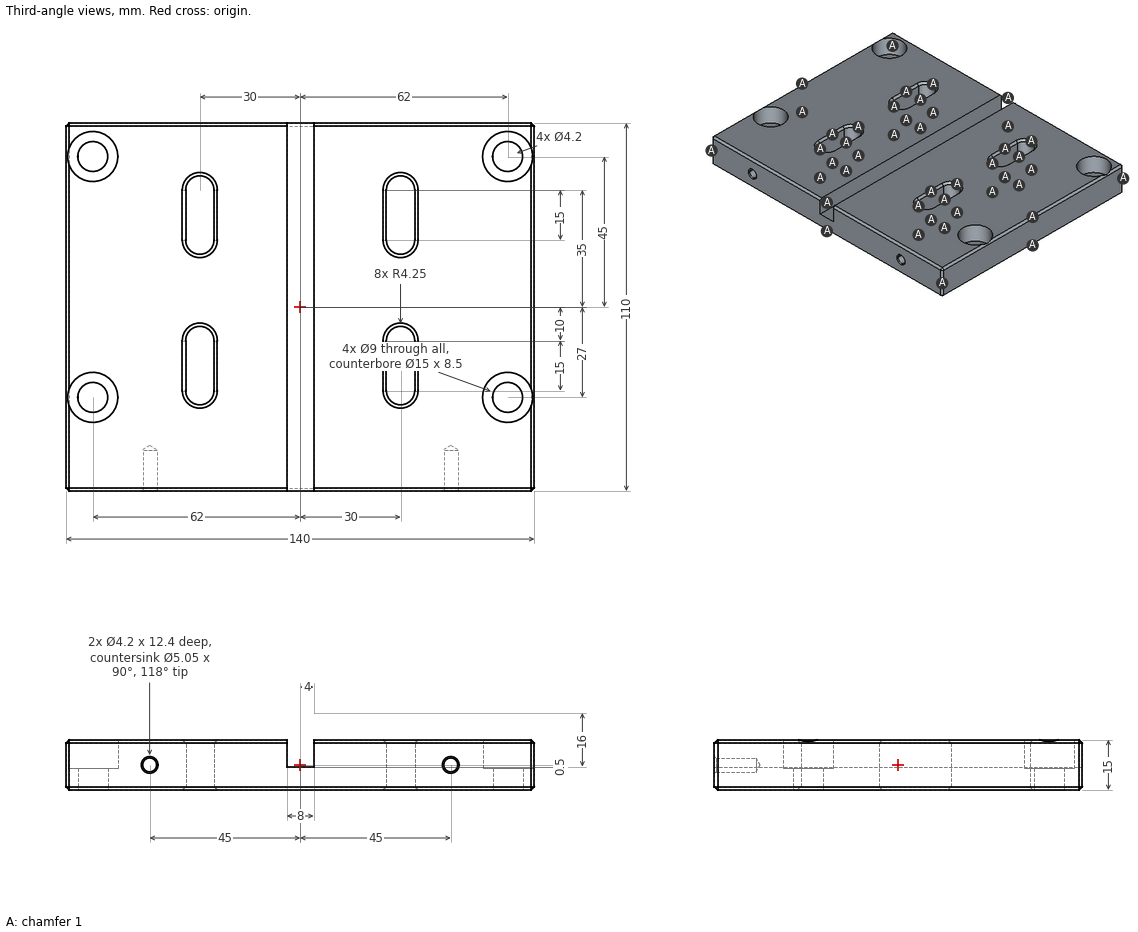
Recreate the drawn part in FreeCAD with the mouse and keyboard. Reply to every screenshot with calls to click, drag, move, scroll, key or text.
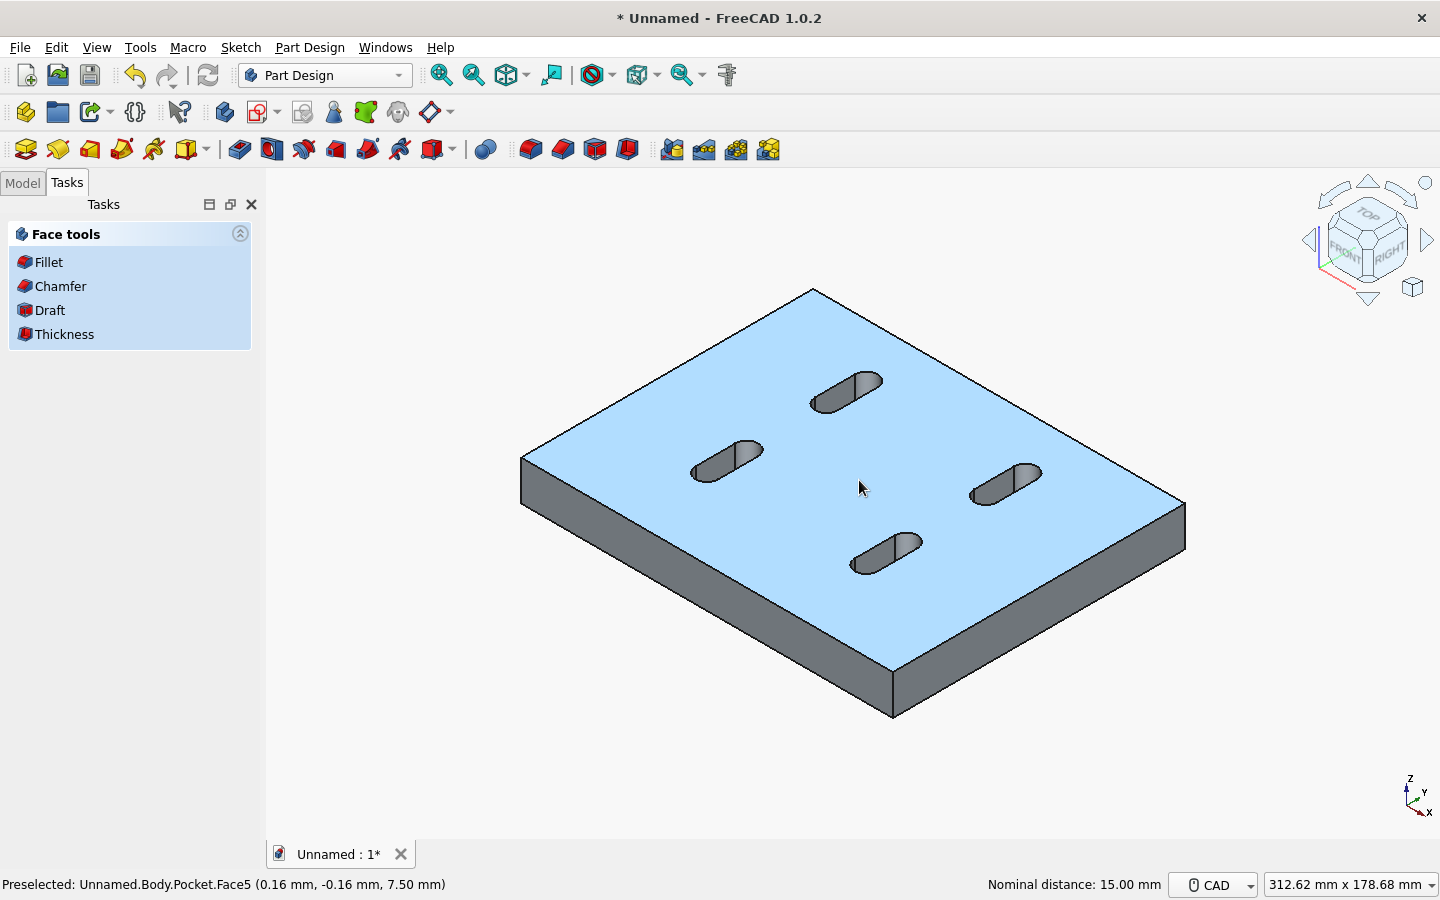
click(893, 694, ctrl)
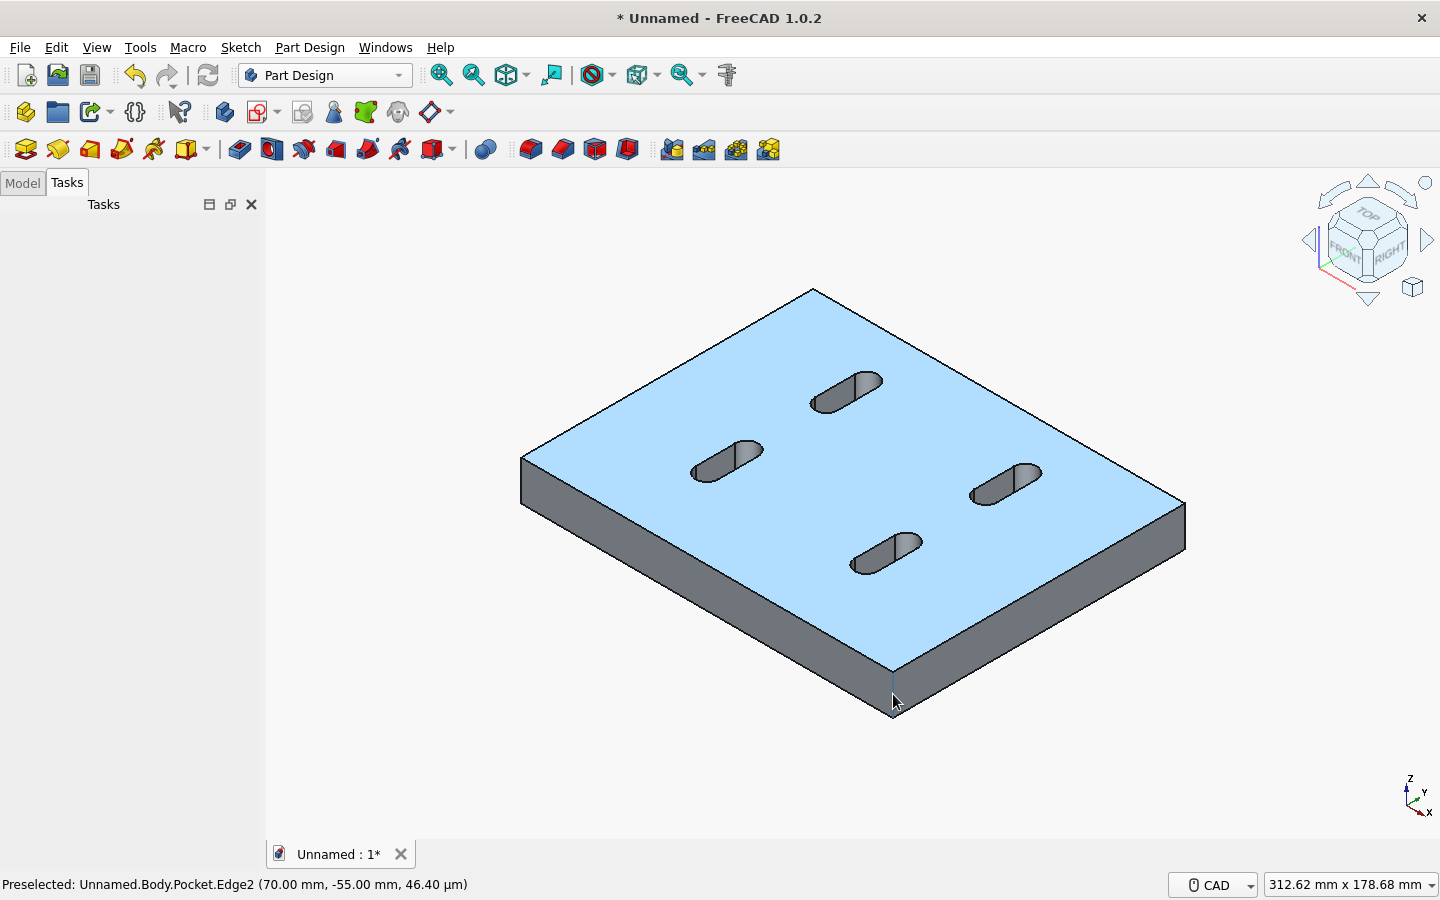
key(2)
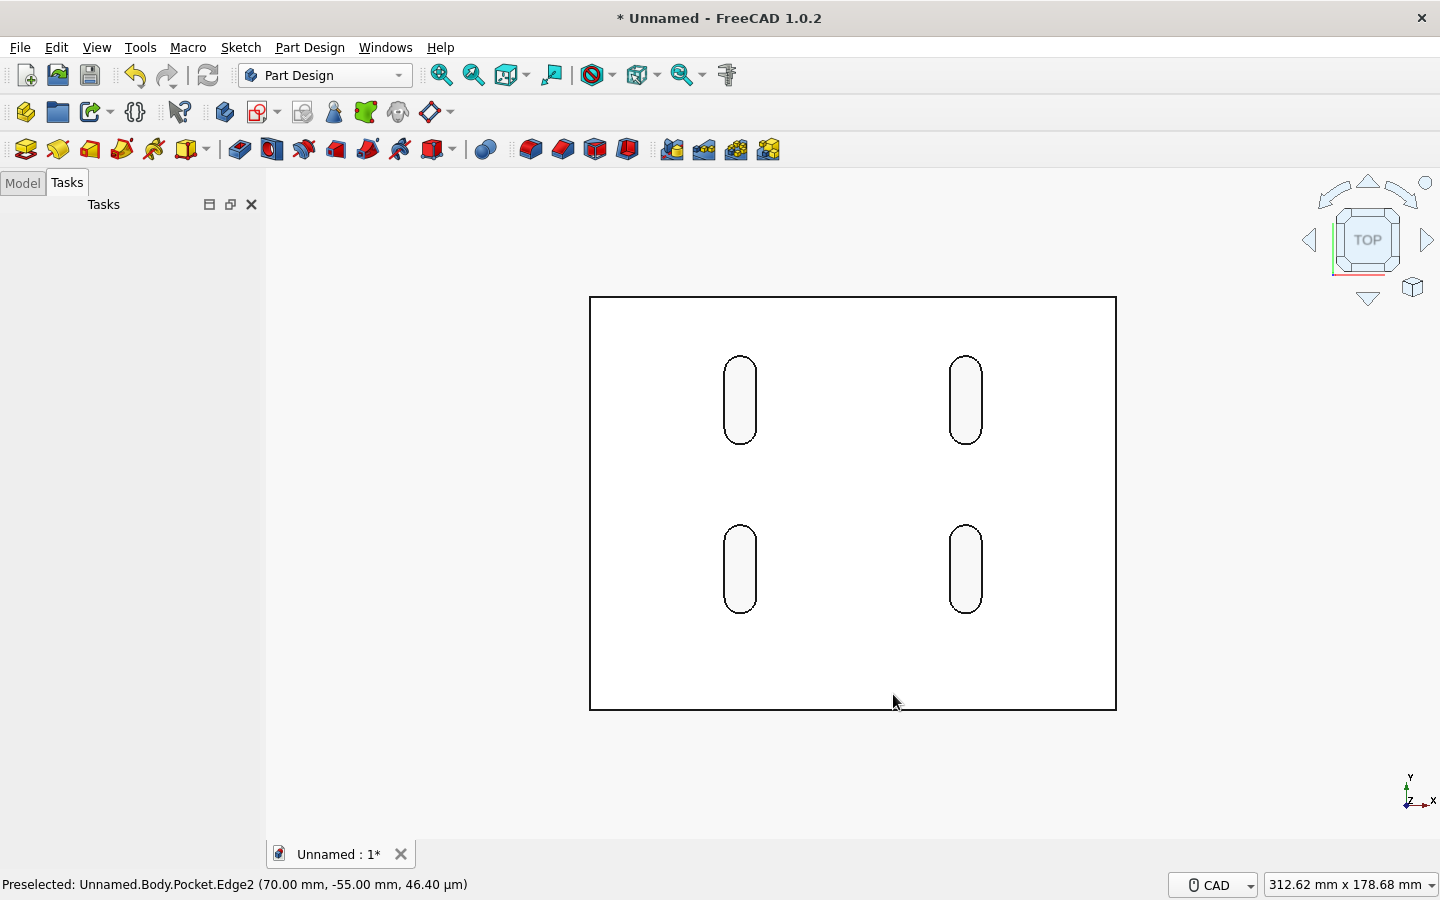
key(1)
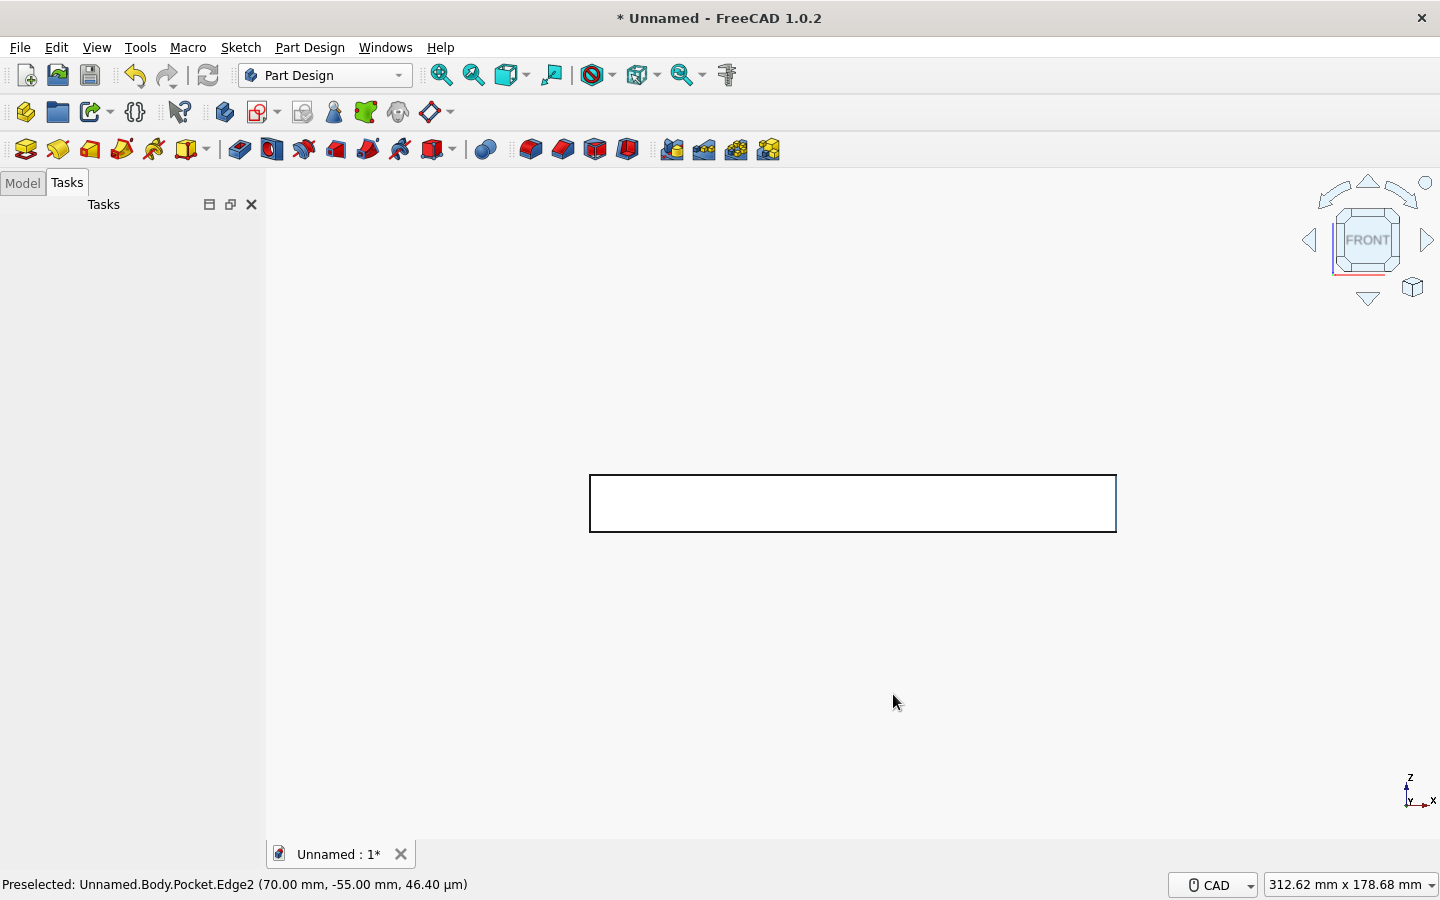
key(v)
key(f)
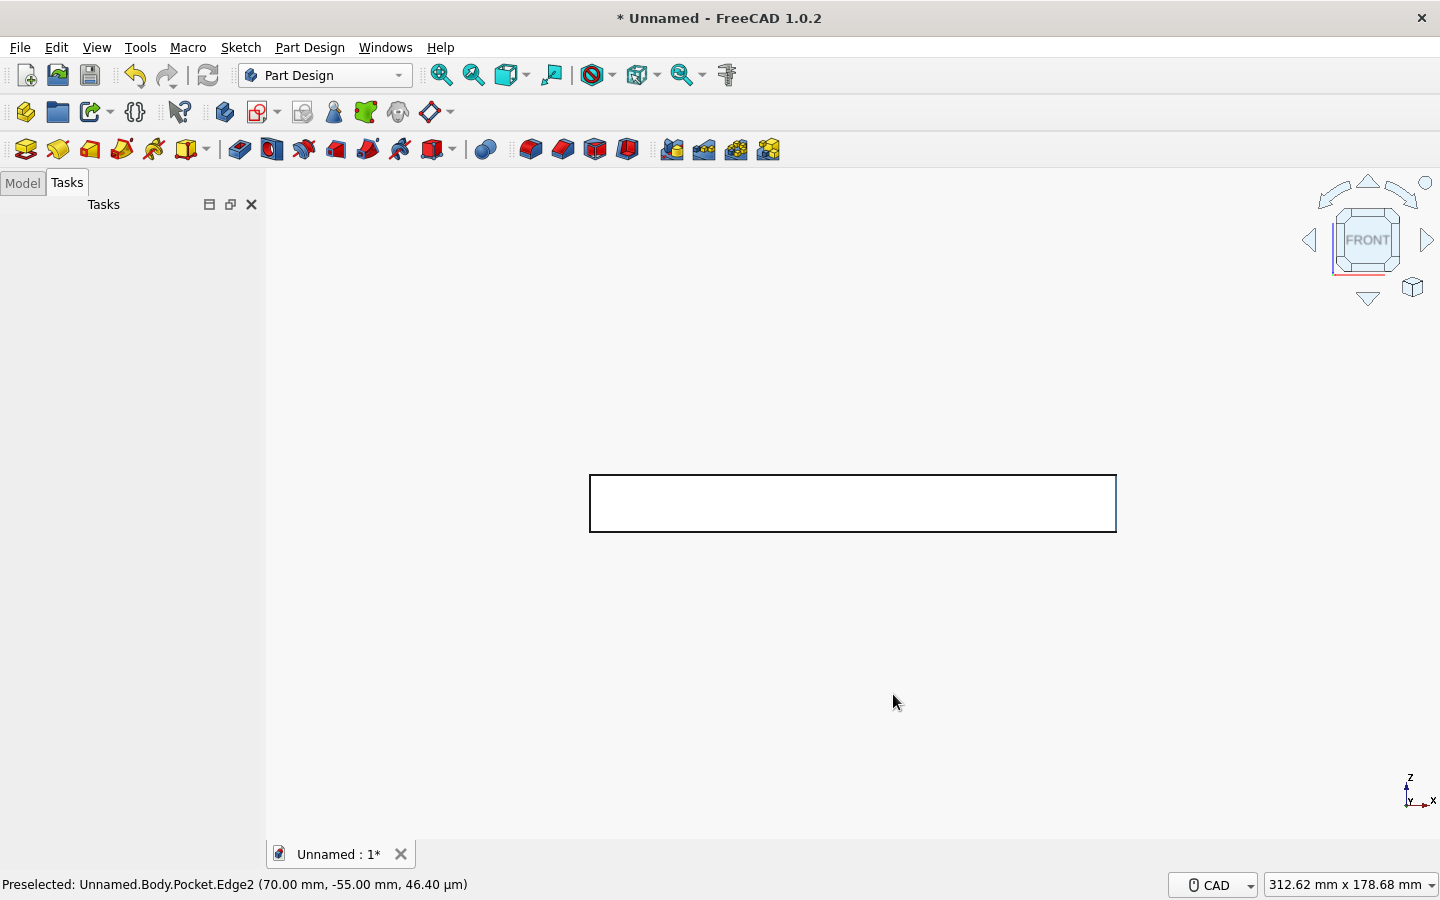
click(590, 503, ctrl)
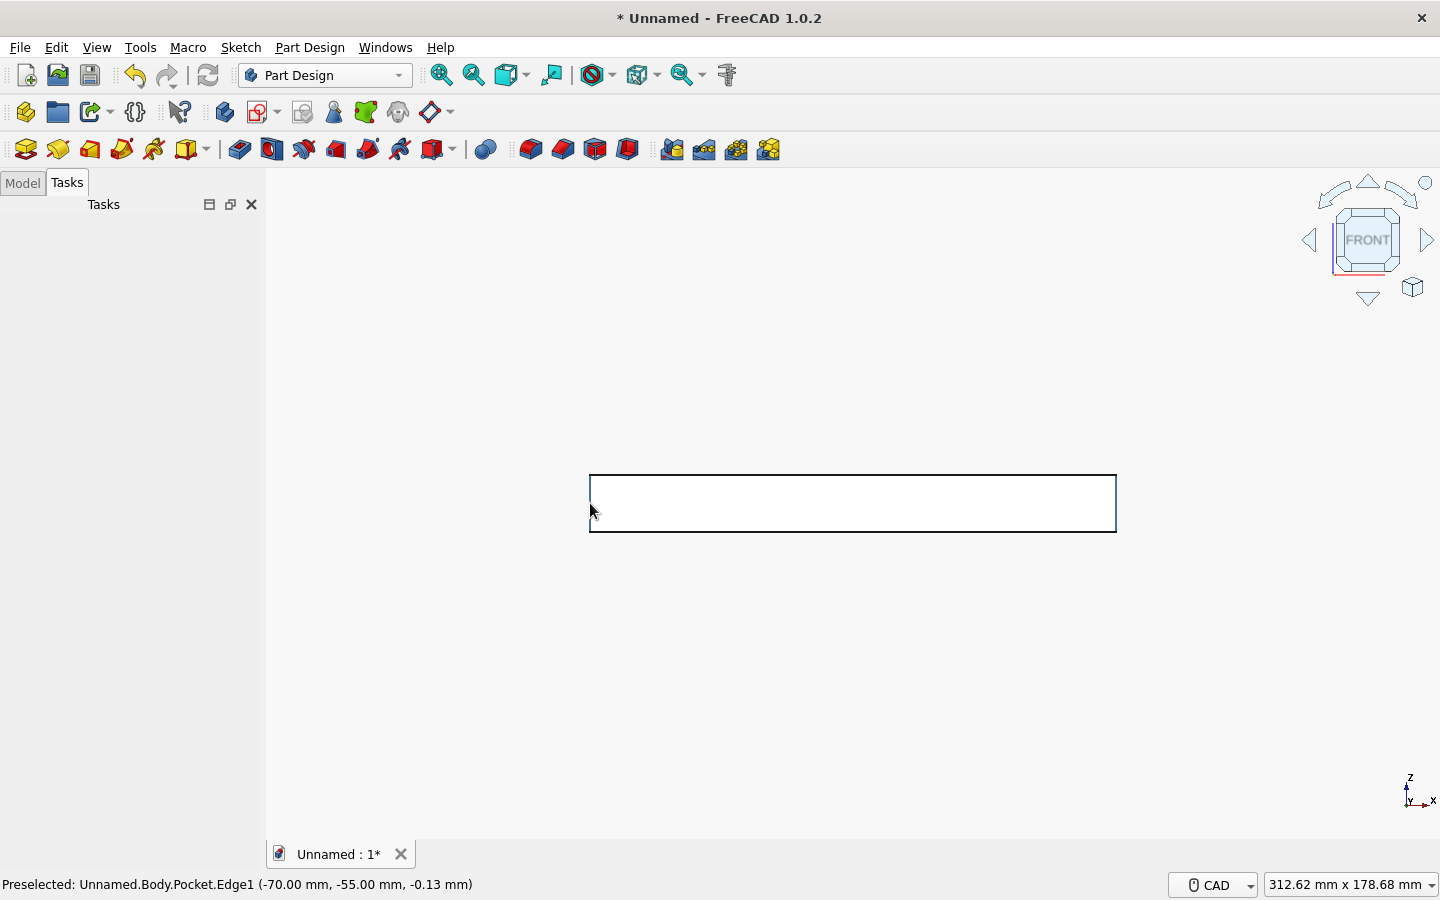
key(3)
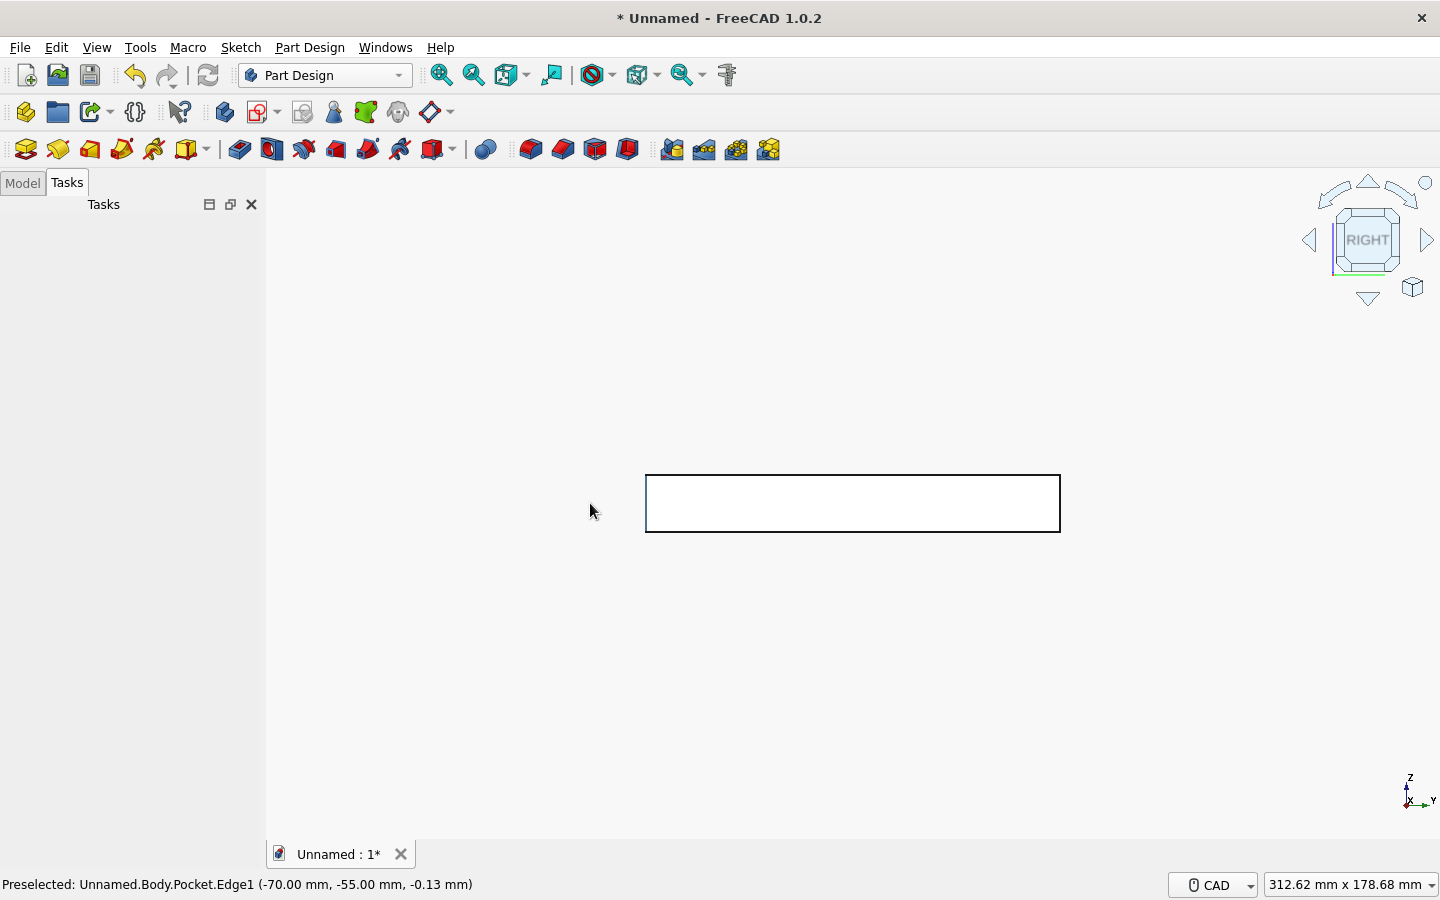
click(442, 76)